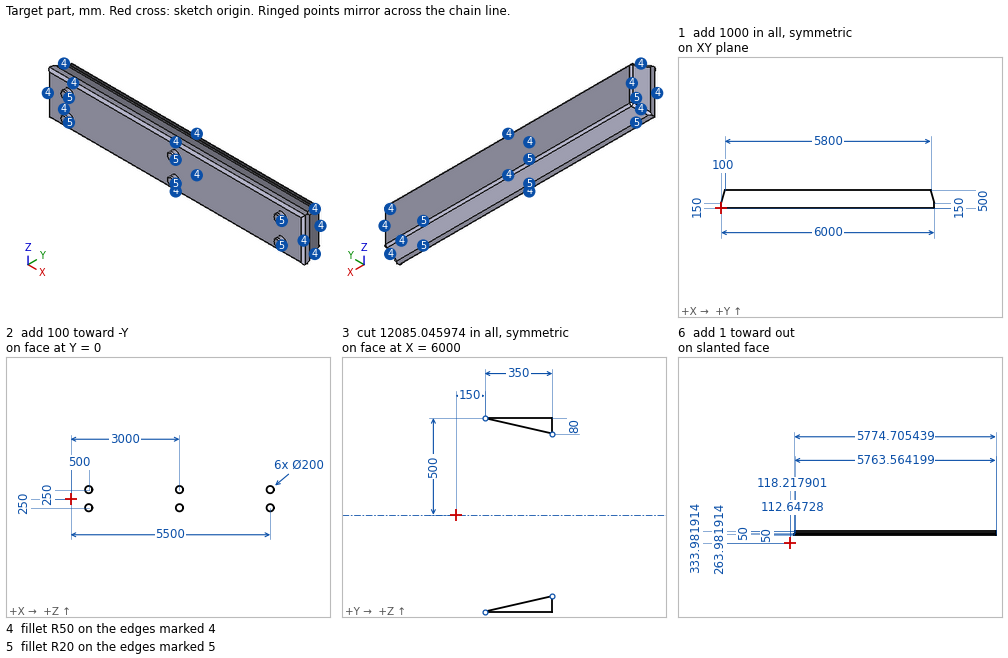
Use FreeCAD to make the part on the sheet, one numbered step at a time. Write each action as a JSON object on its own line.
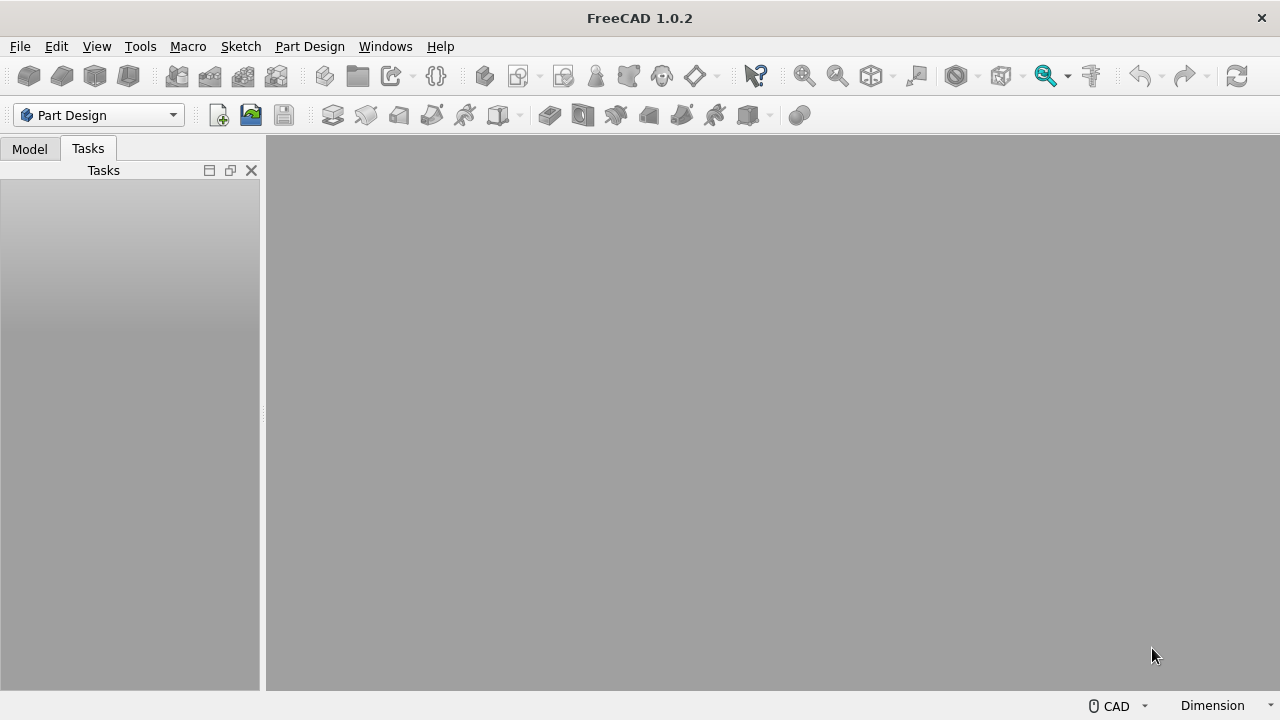
{"action": "left_click", "coordinate": [218, 116]}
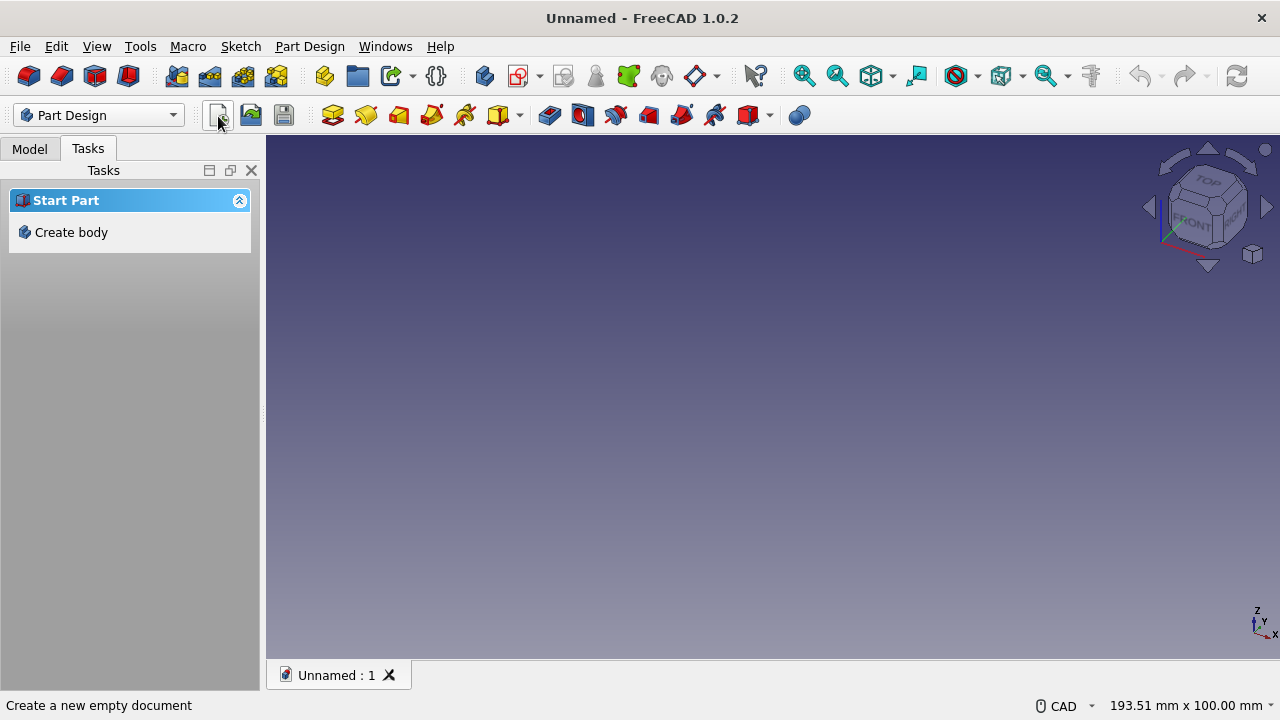
{"action": "left_click", "coordinate": [518, 76]}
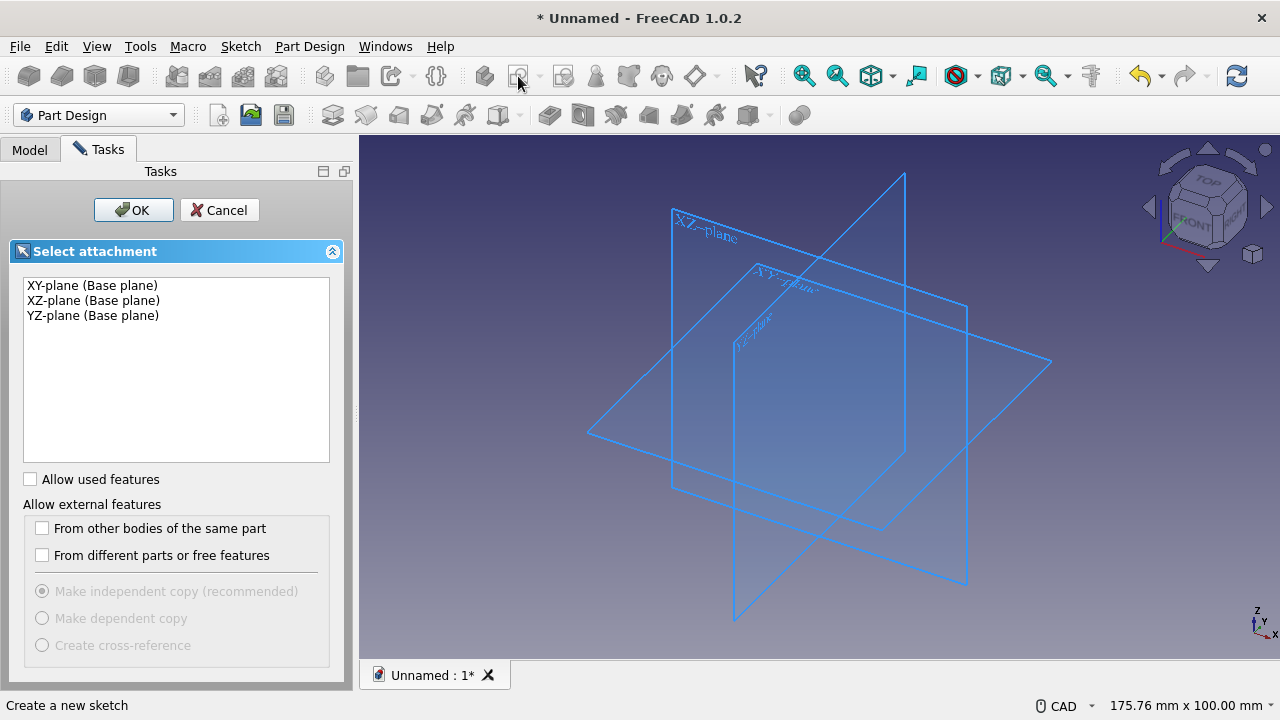
{"action": "left_click", "coordinate": [84, 286]}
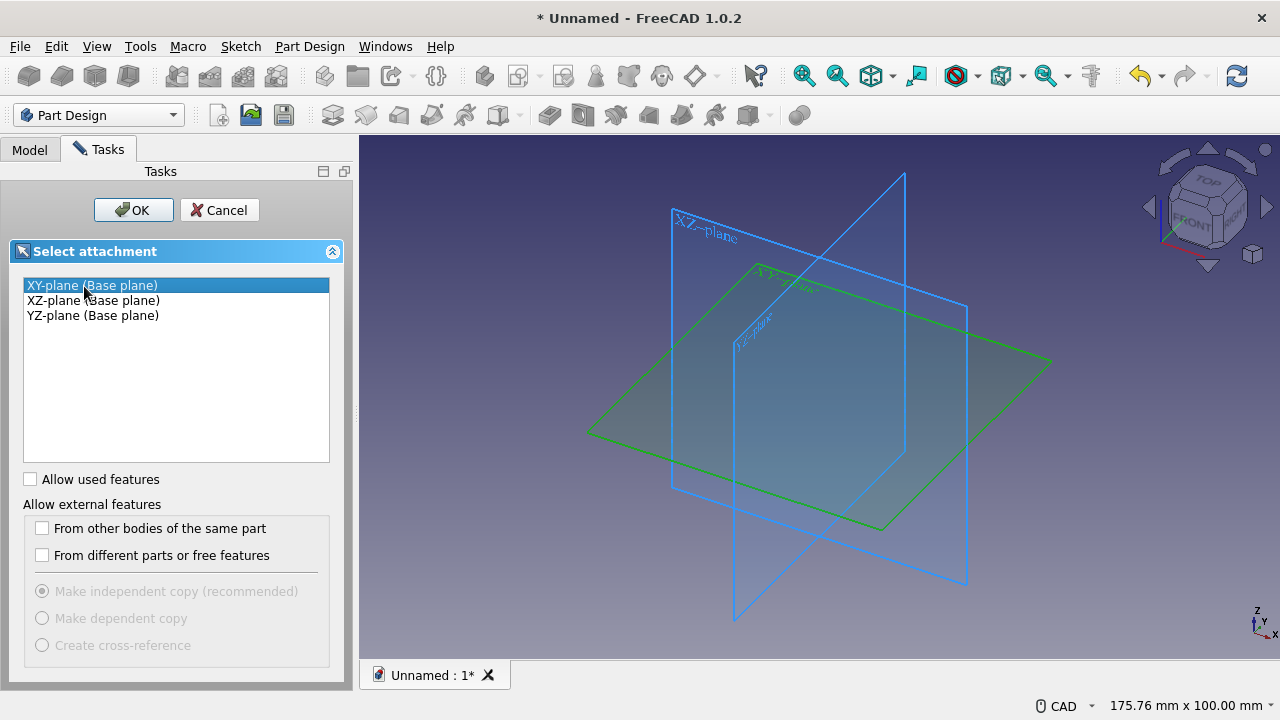
{"action": "left_click", "coordinate": [134, 210]}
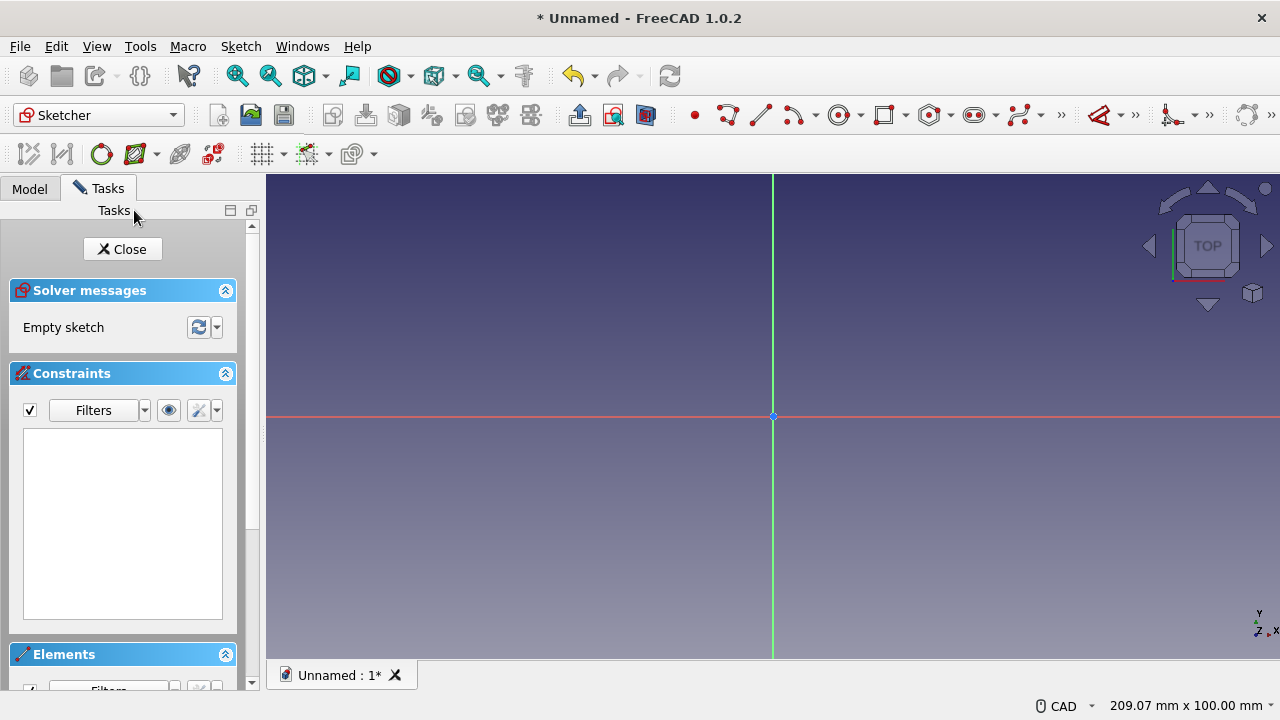
{"action": "scroll", "coordinate": [704, 416], "scroll_direction": "down", "scroll_amount": 15}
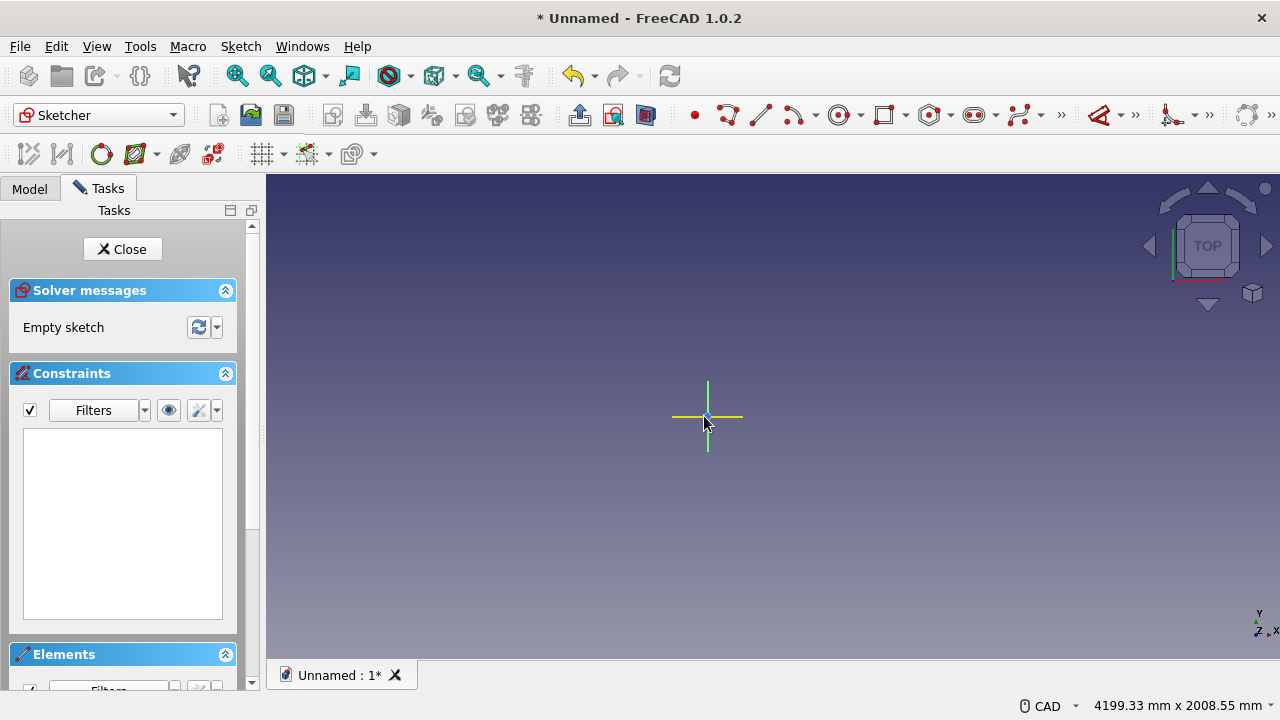
{"action": "scroll", "coordinate": [294, 452], "scroll_direction": "down", "scroll_amount": 5}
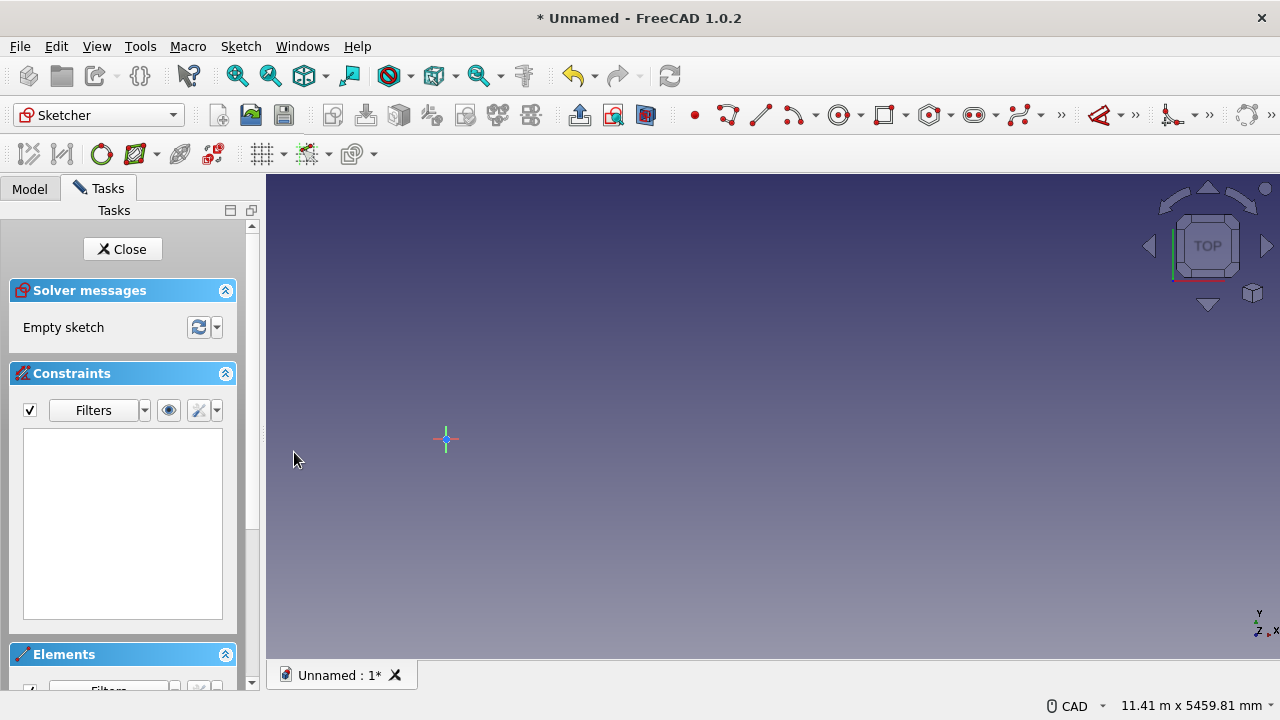
{"action": "left_click", "coordinate": [728, 116]}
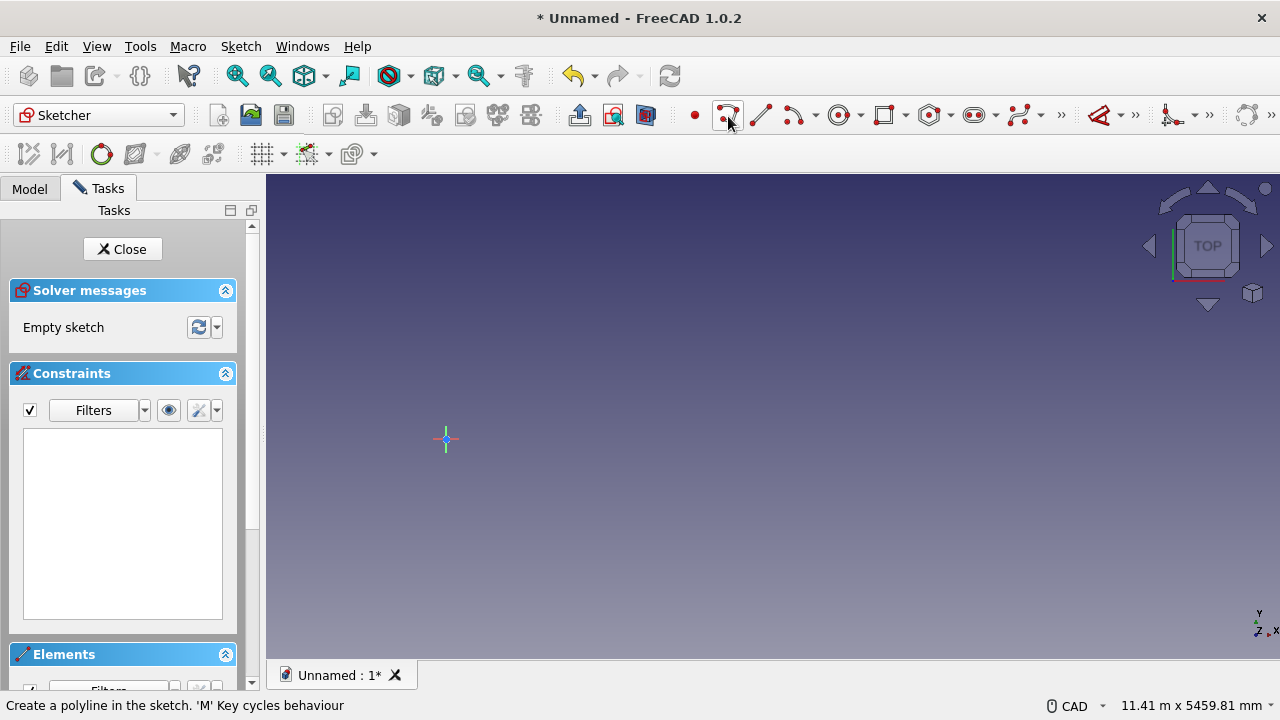
{"action": "left_click", "coordinate": [446, 439]}
{"action": "left_click", "coordinate": [979, 430]}
{"action": "left_click", "coordinate": [979, 426]}
{"action": "left_click", "coordinate": [970, 395]}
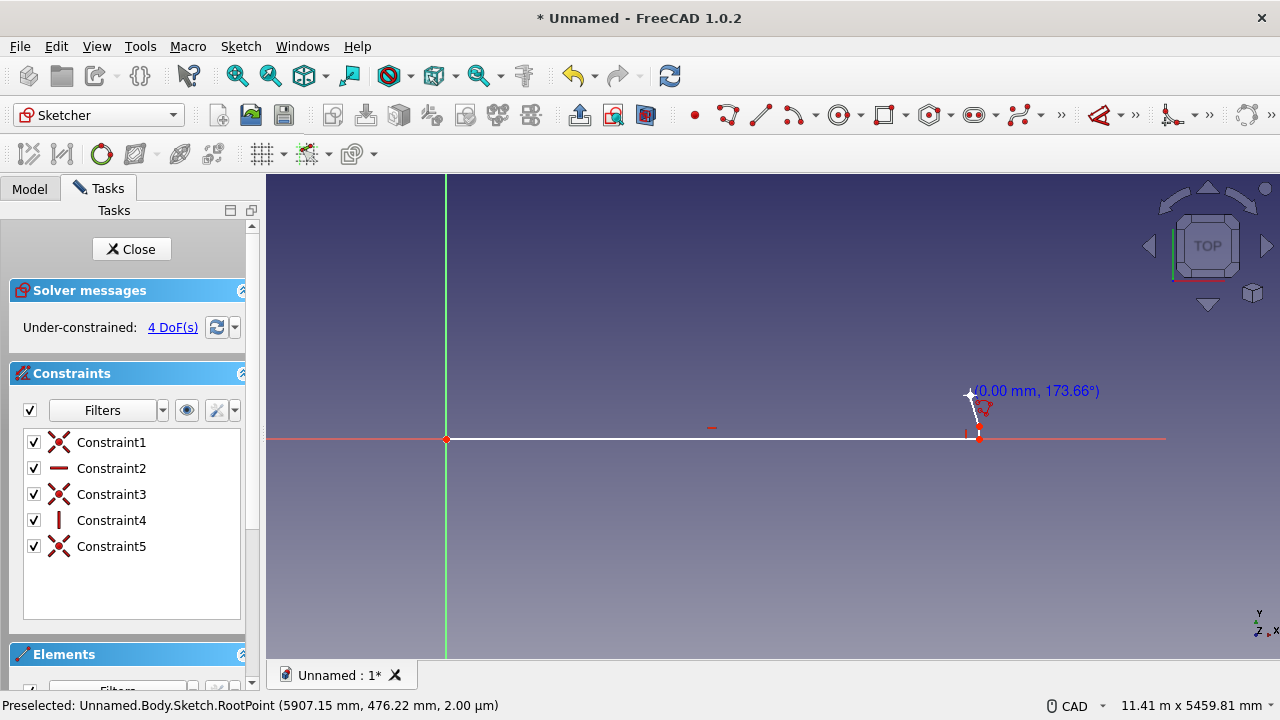
{"action": "scroll", "coordinate": [455, 395], "scroll_direction": "up", "scroll_amount": 3}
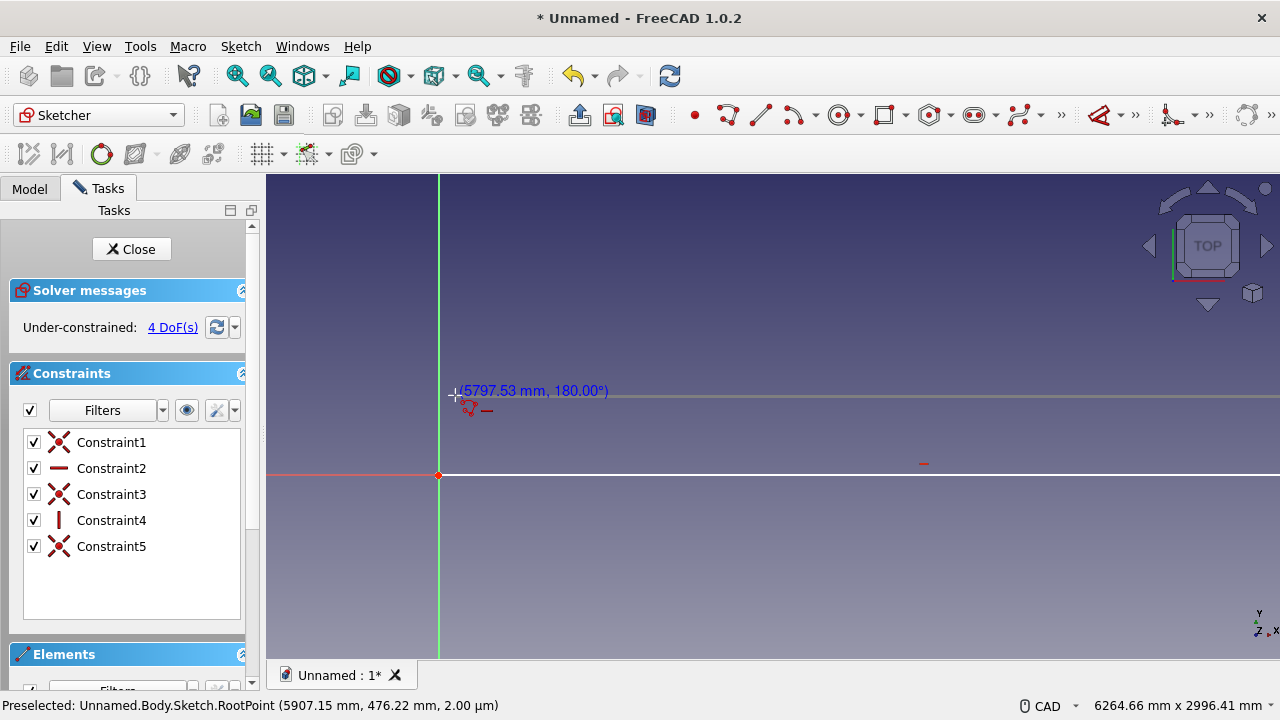
{"action": "left_click", "coordinate": [455, 395]}
{"action": "left_click", "coordinate": [448, 451]}
{"action": "left_click", "coordinate": [439, 475]}
{"action": "key", "text": "Escape"}
{"action": "key", "text": "Escape"}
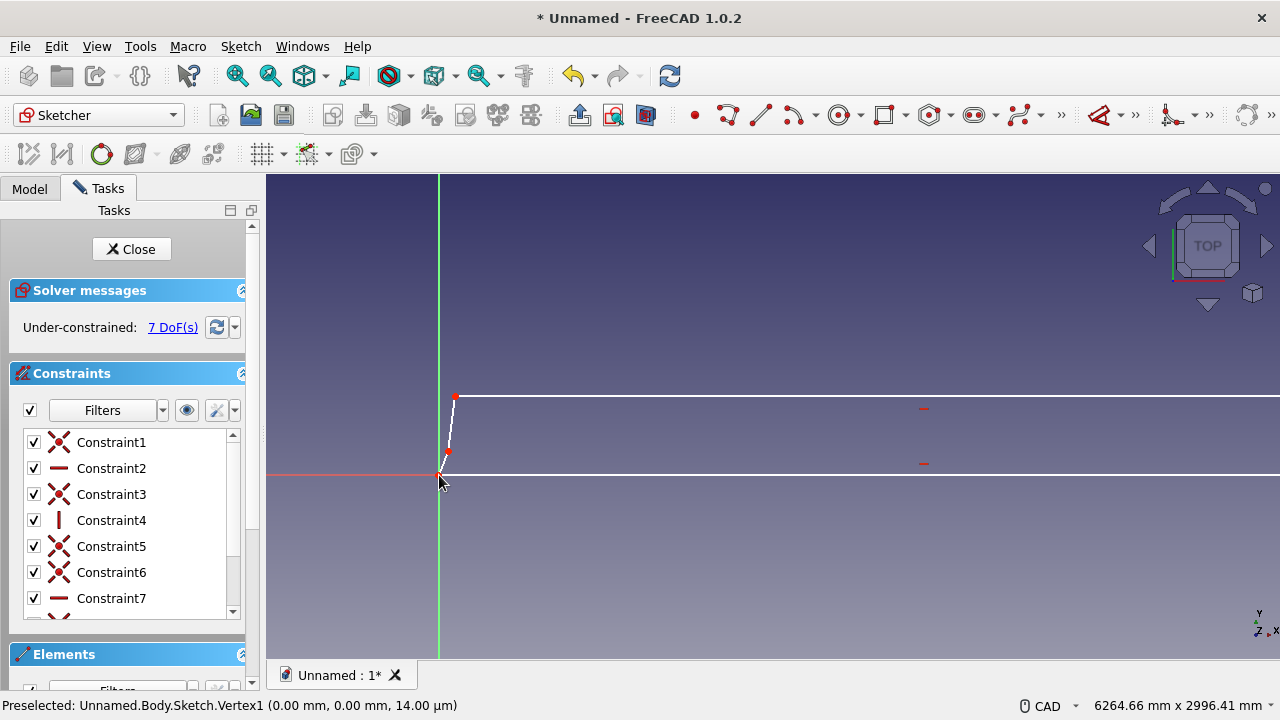
{"action": "scroll", "coordinate": [443, 466], "scroll_direction": "up", "scroll_amount": 2}